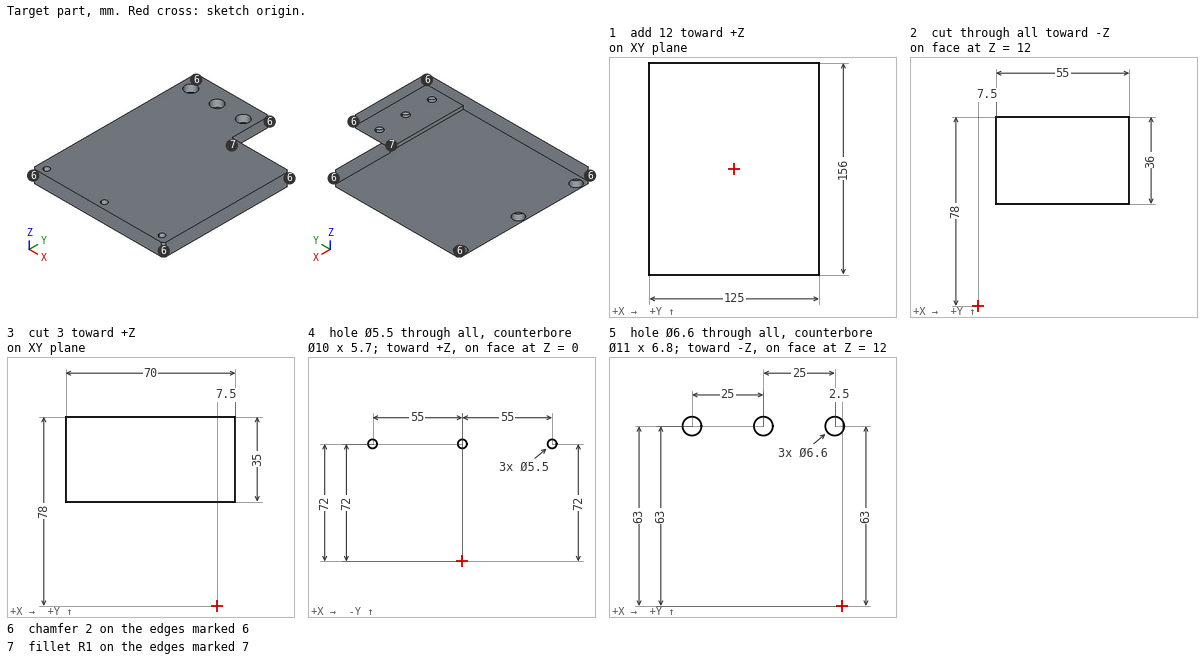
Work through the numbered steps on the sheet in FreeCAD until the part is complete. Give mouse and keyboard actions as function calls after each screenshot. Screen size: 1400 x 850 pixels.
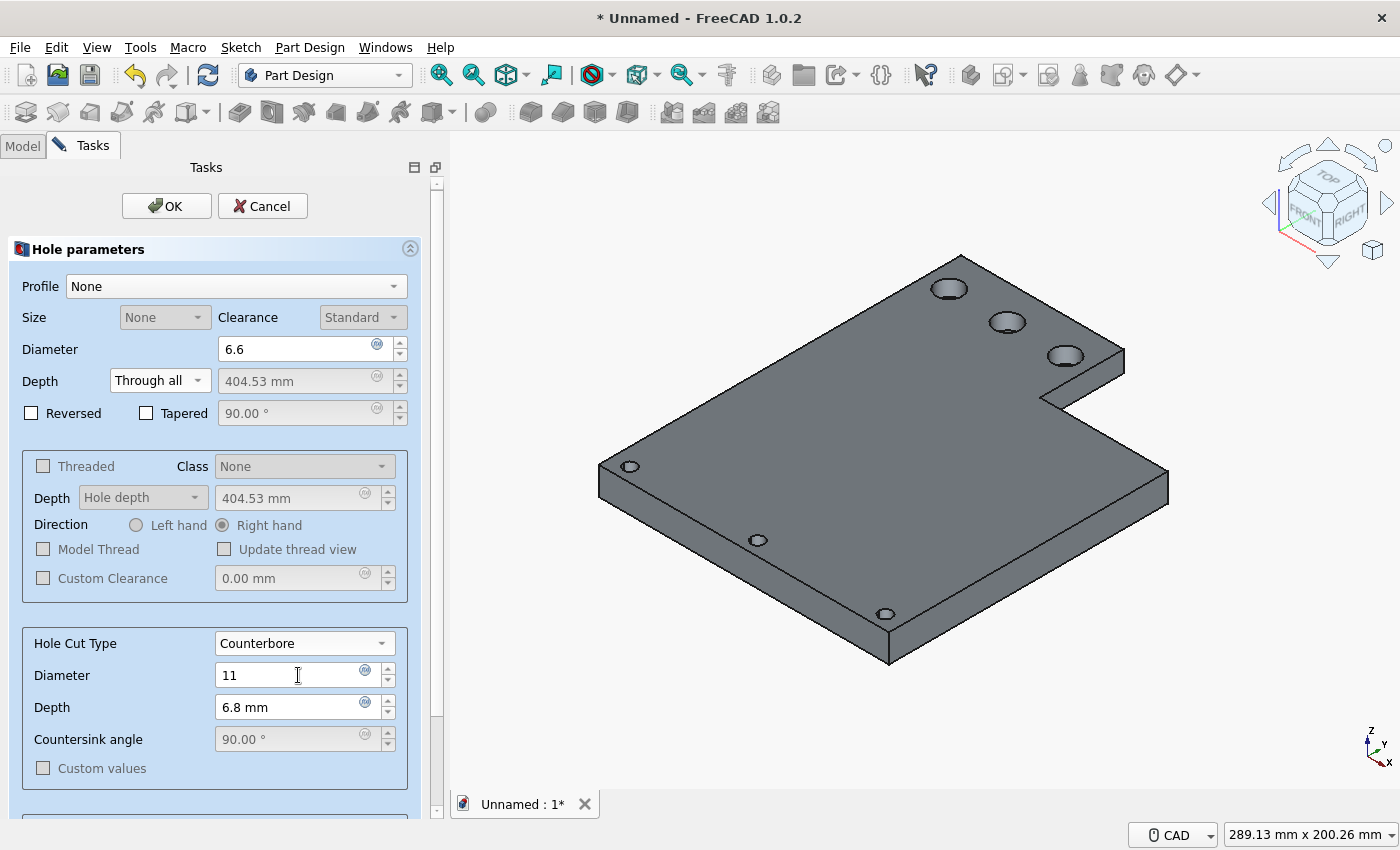
click(167, 206)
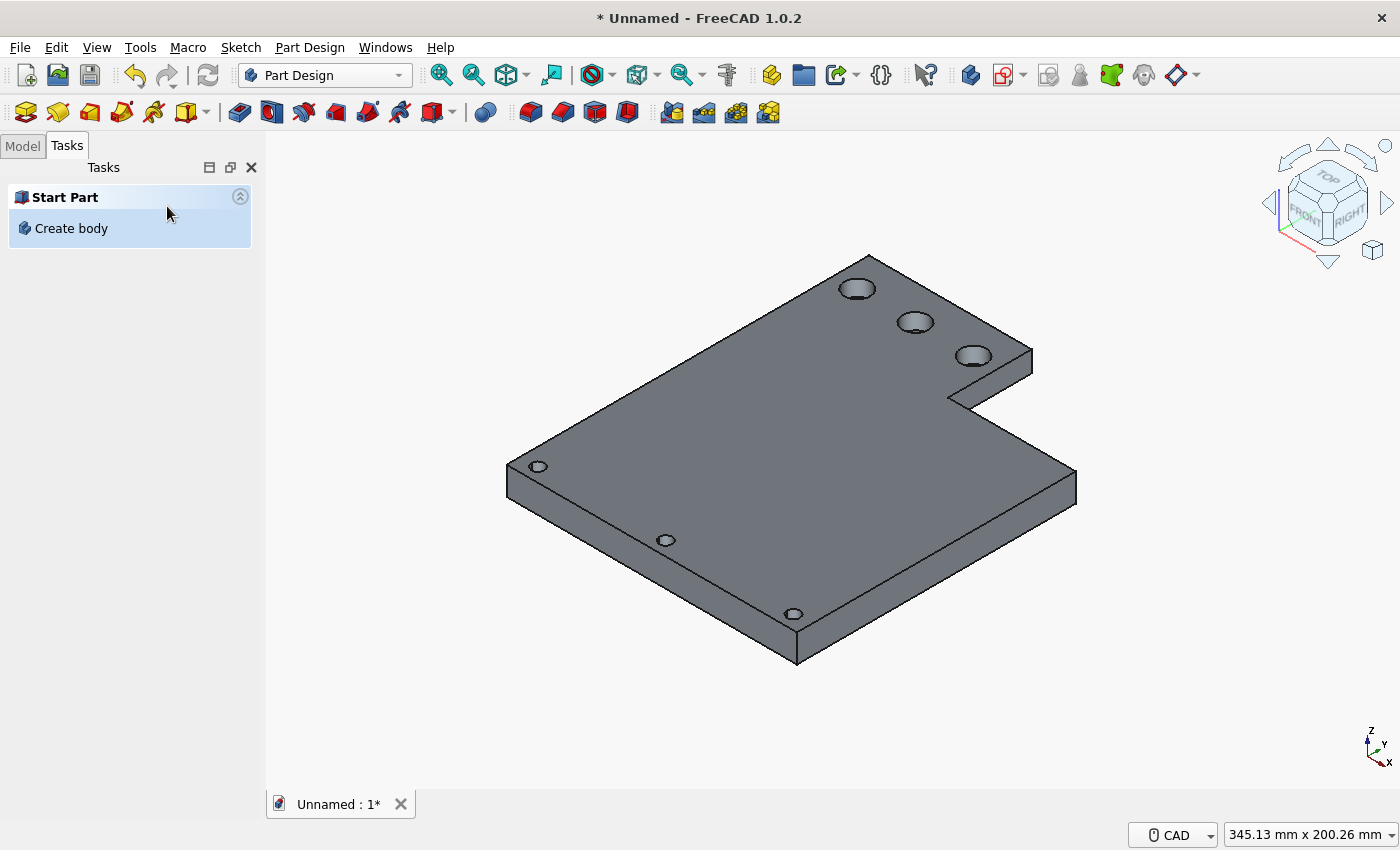
click(797, 647)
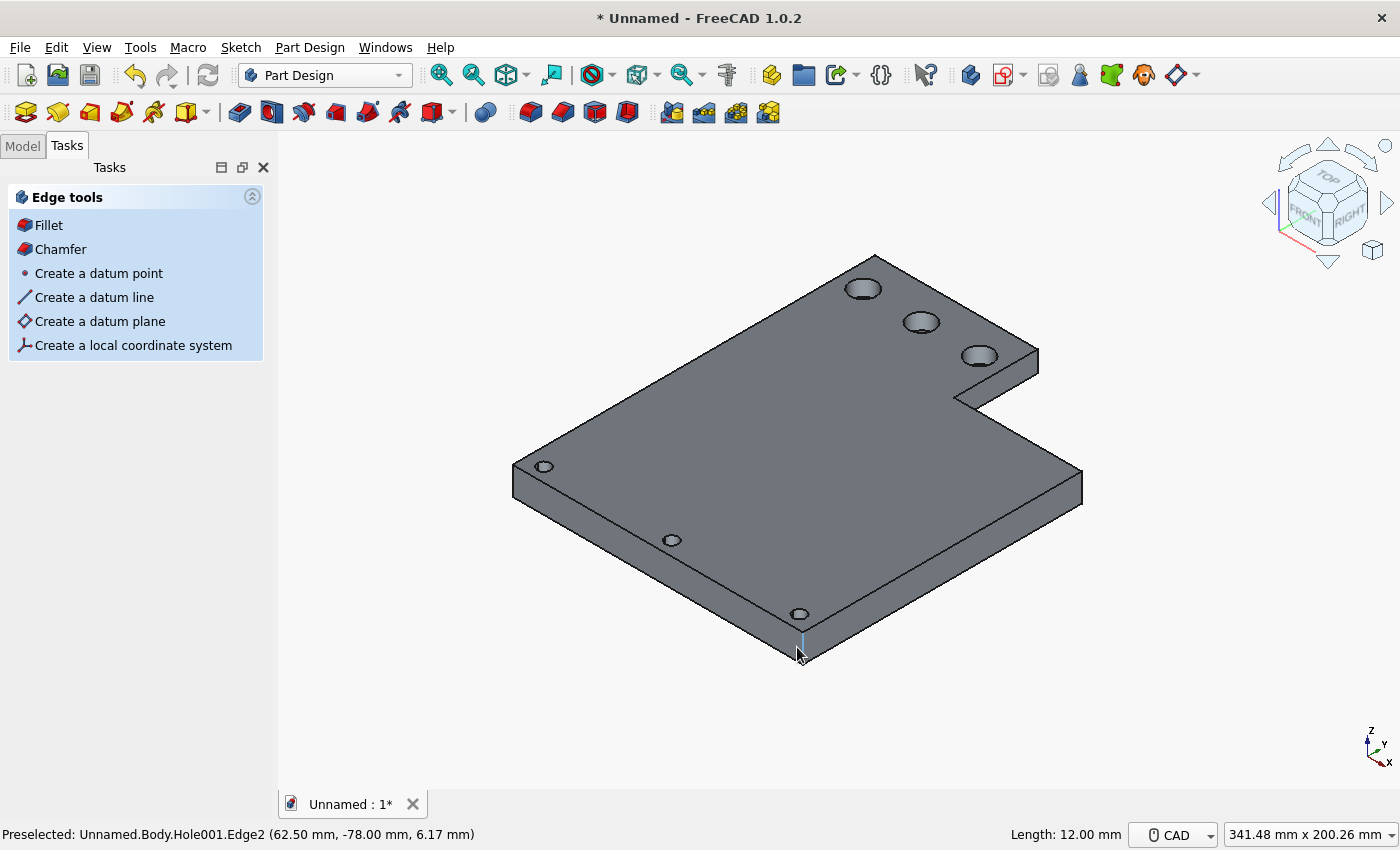
key(2)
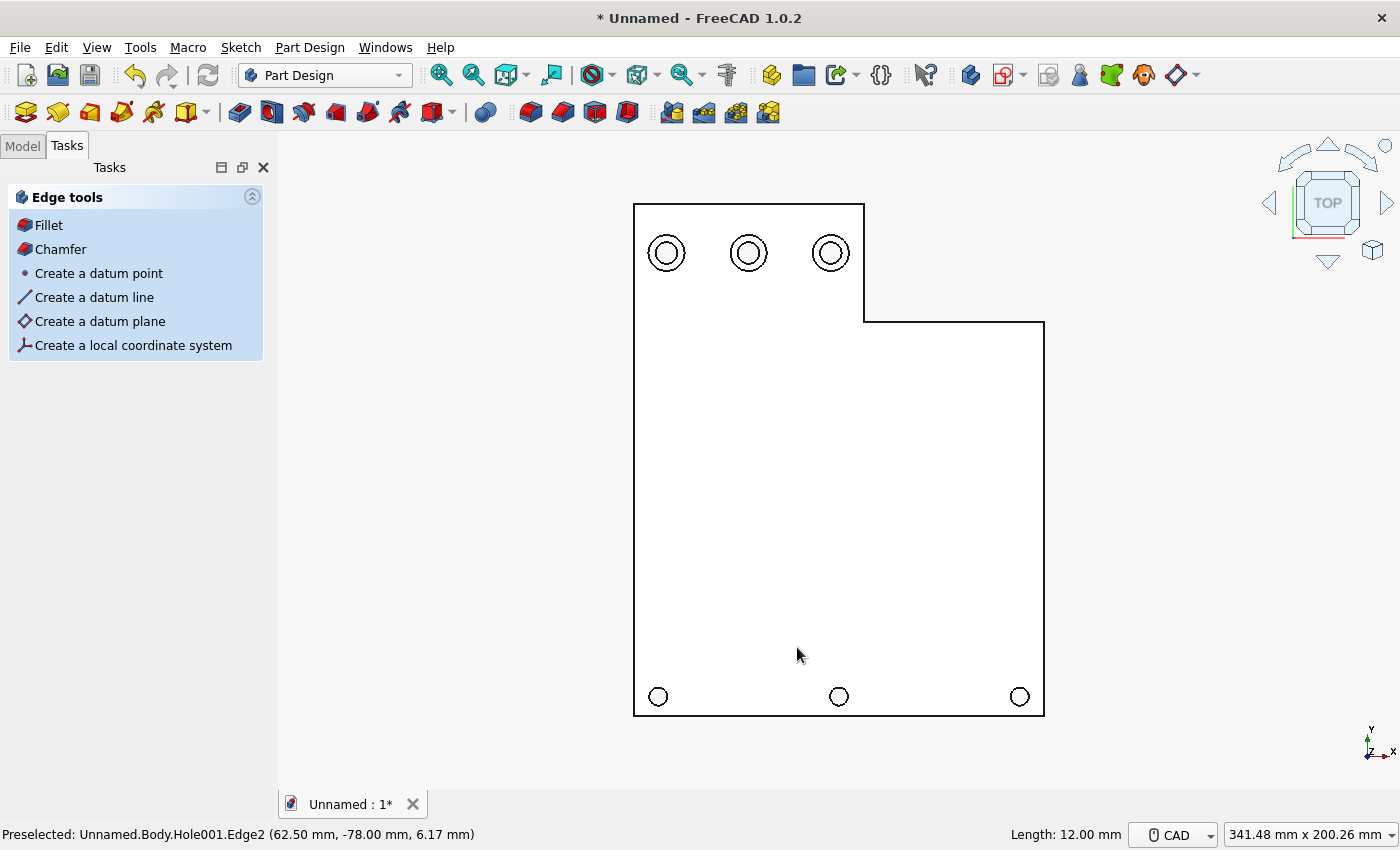
key(0)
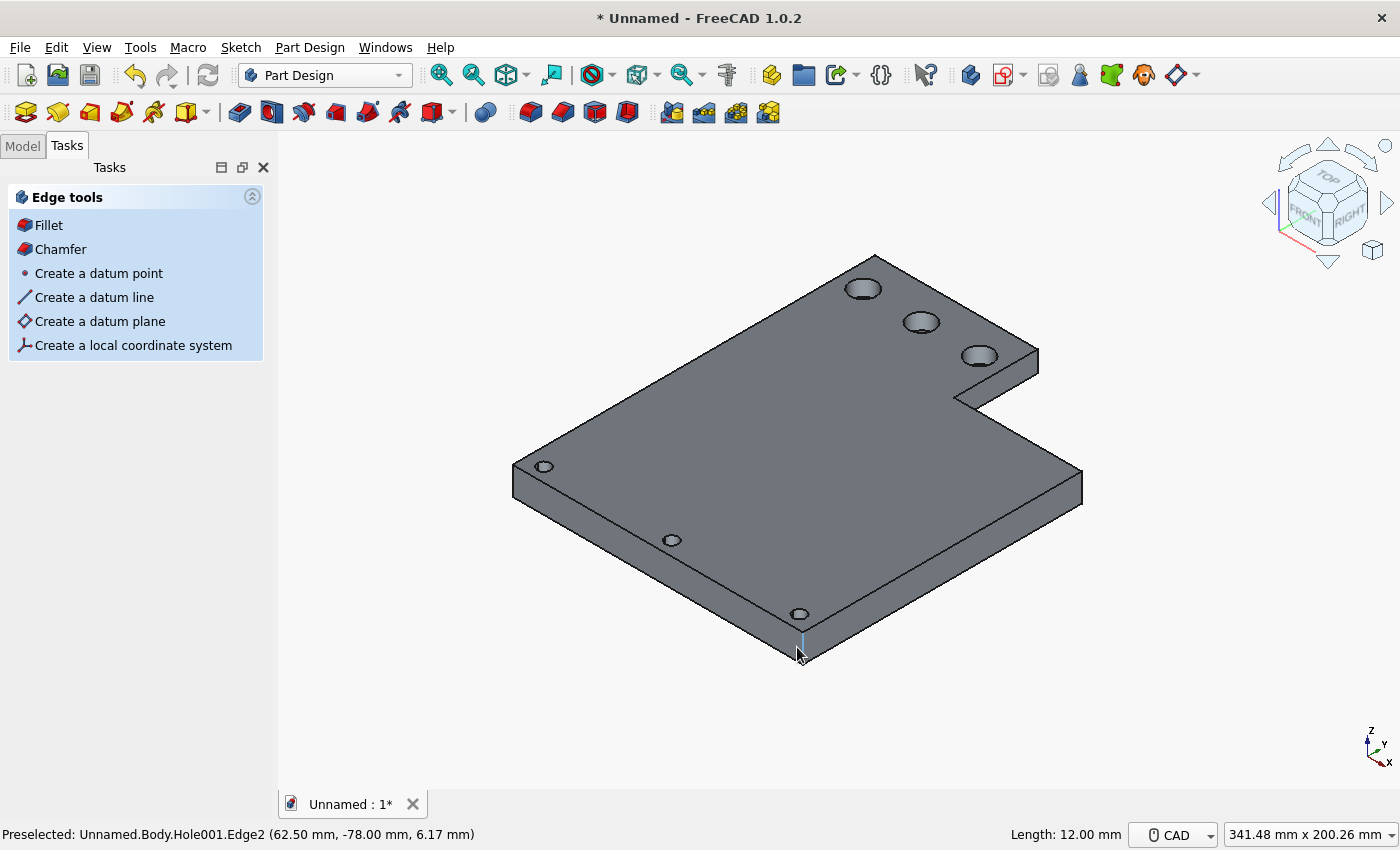
key(1)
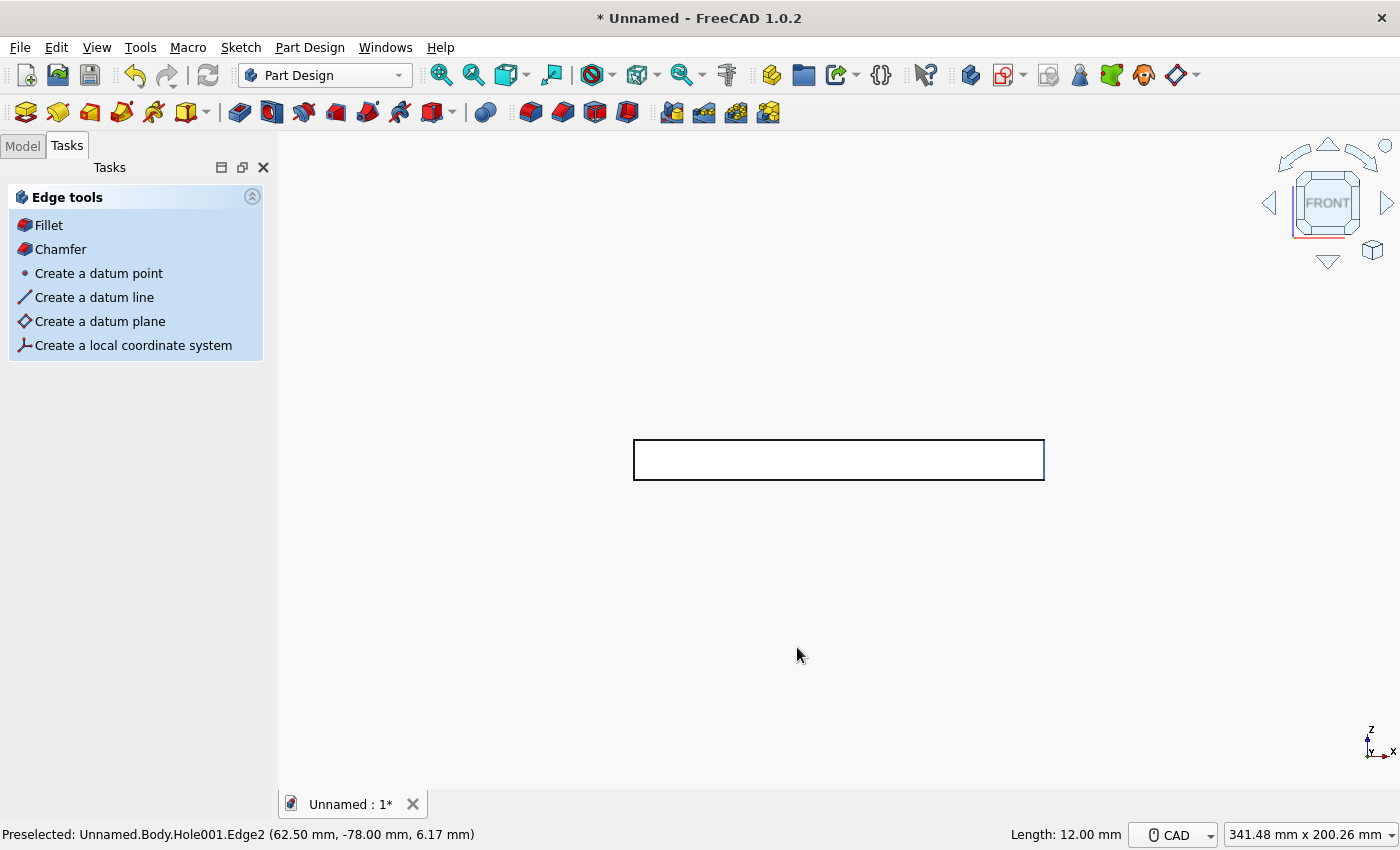
click(442, 76)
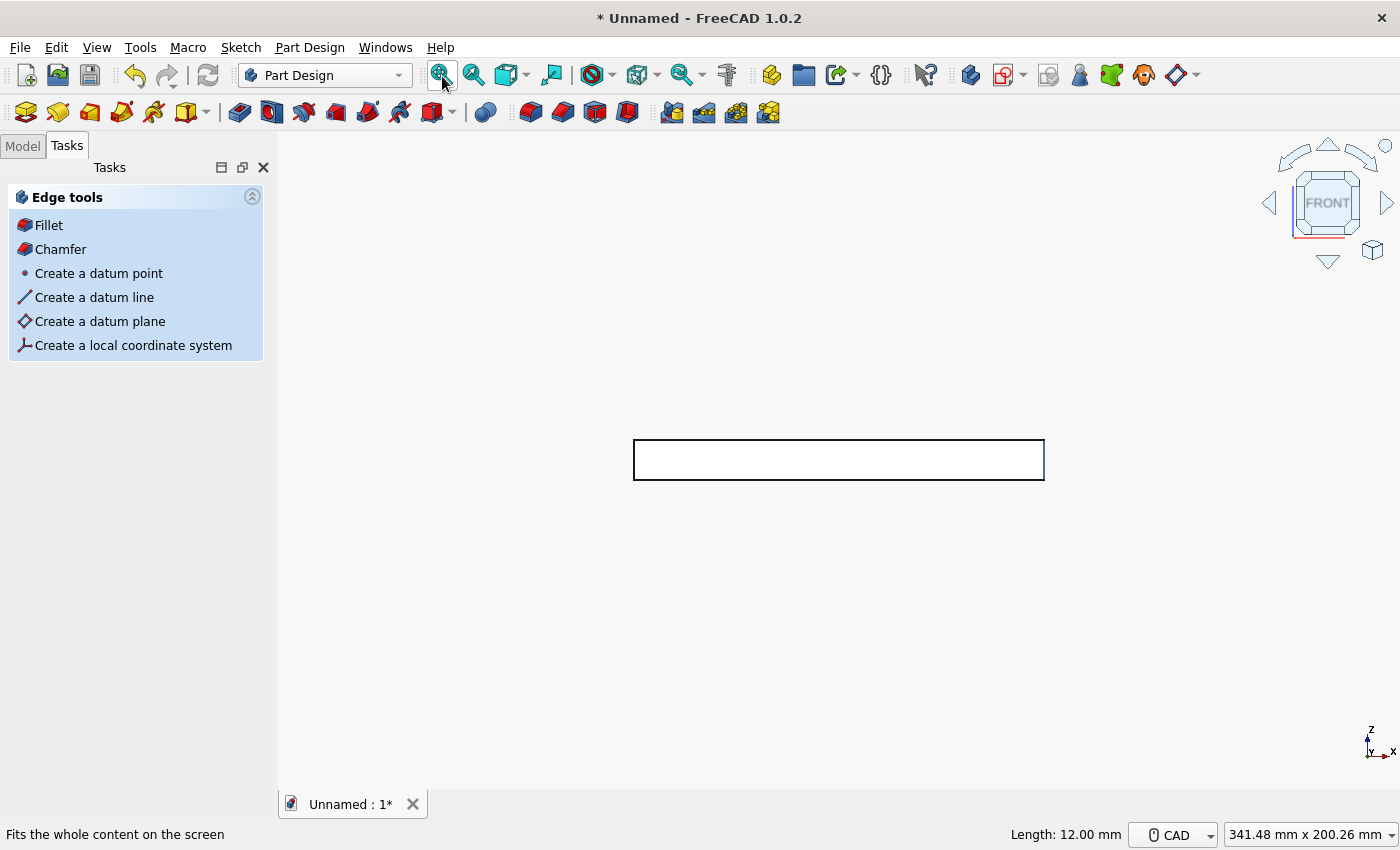
click(634, 459, ctrl)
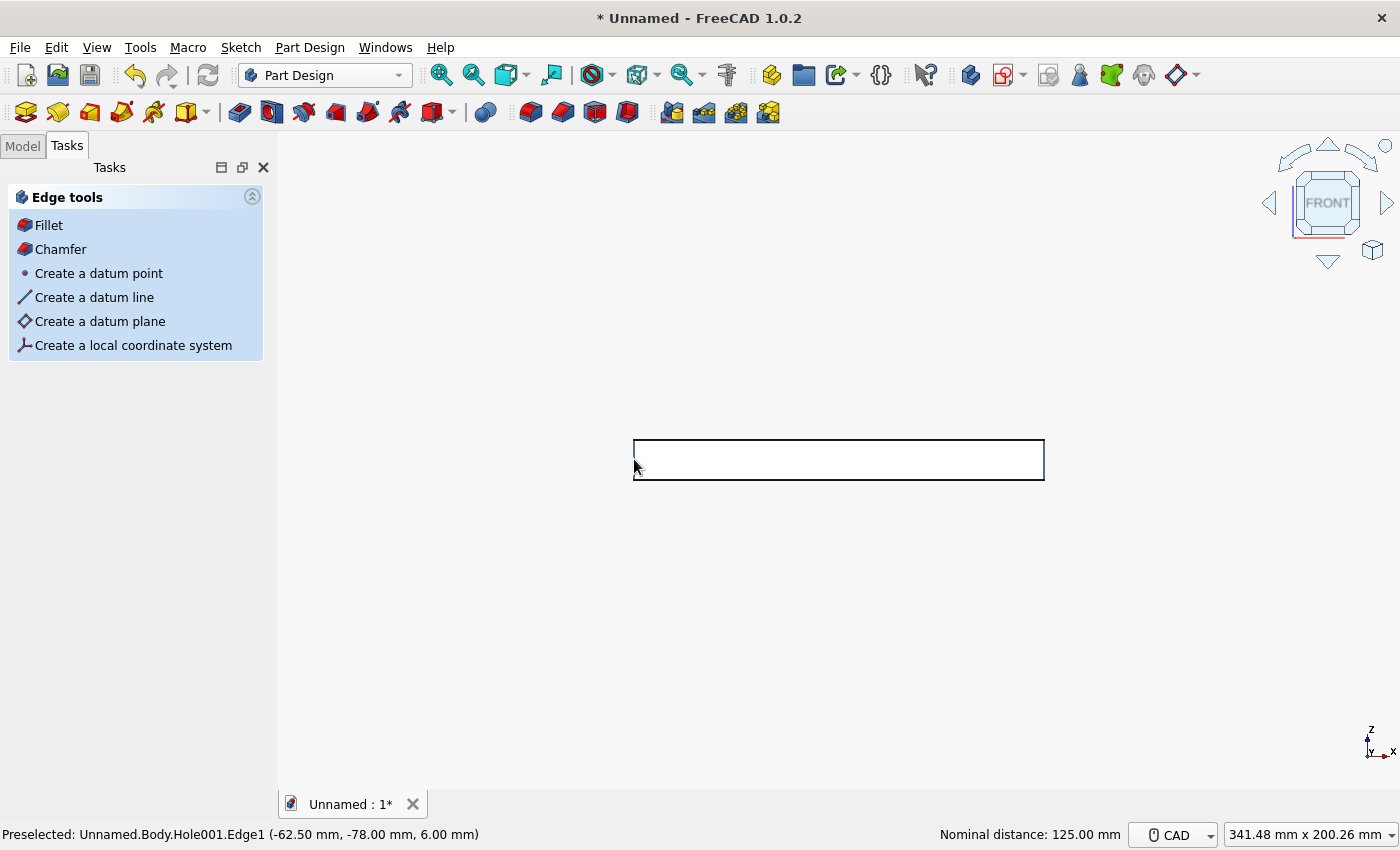
key(3)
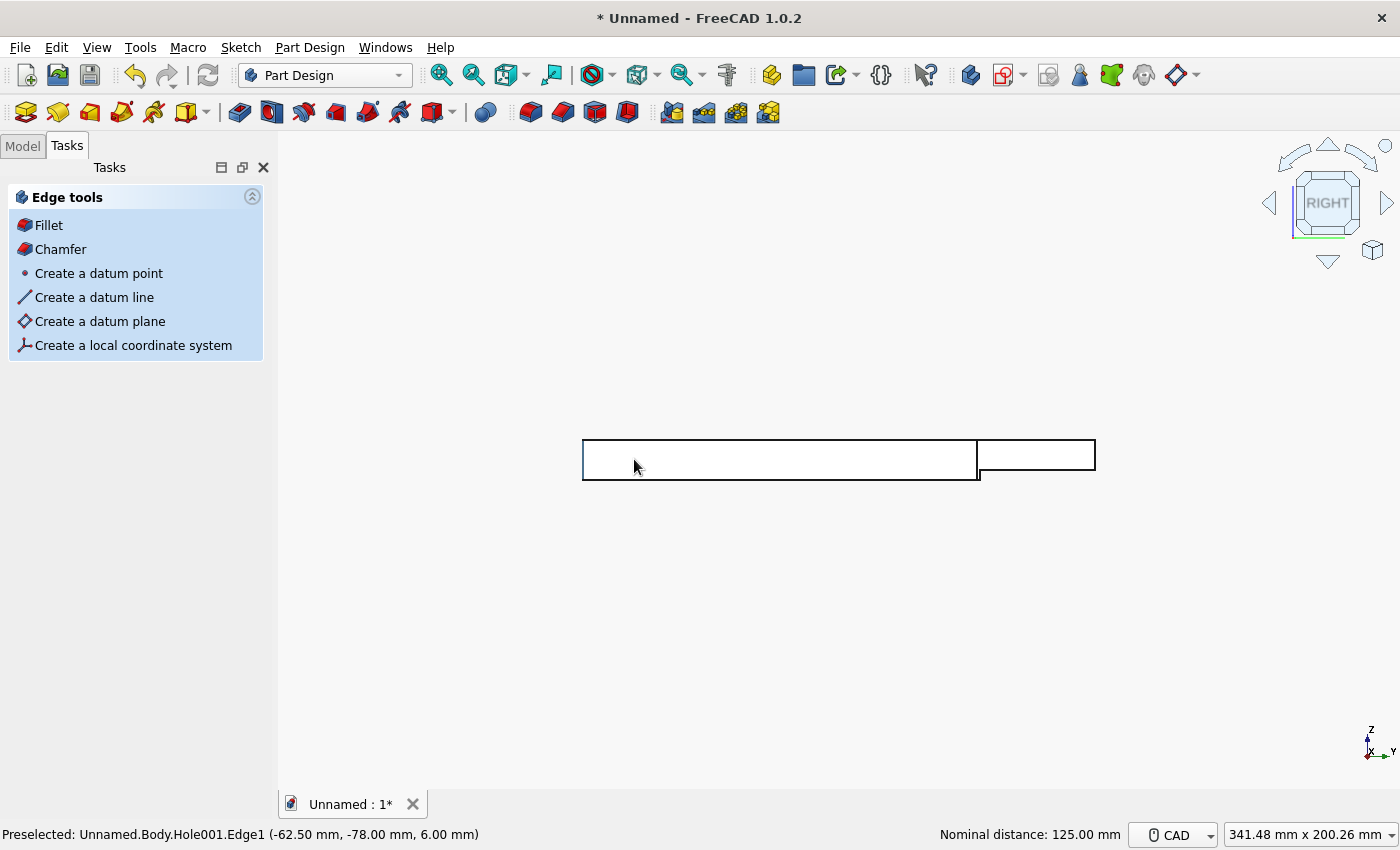
click(977, 459, ctrl)